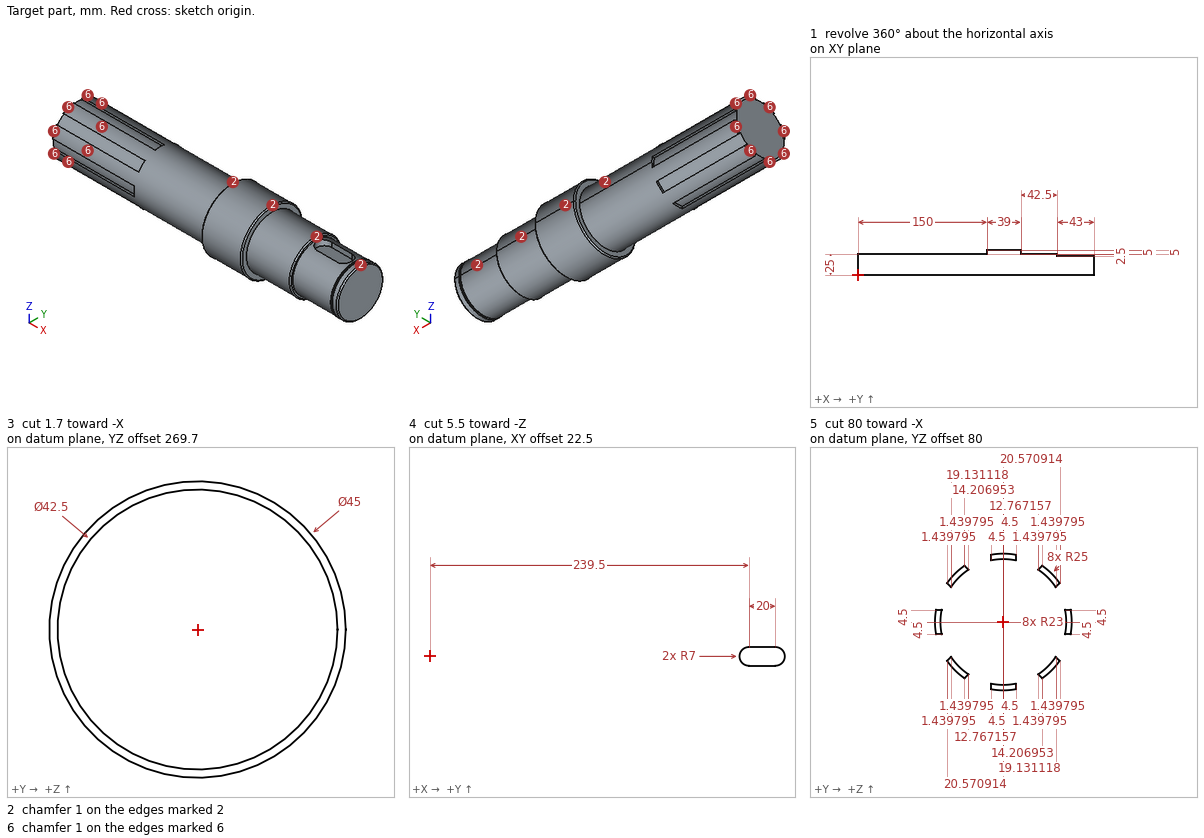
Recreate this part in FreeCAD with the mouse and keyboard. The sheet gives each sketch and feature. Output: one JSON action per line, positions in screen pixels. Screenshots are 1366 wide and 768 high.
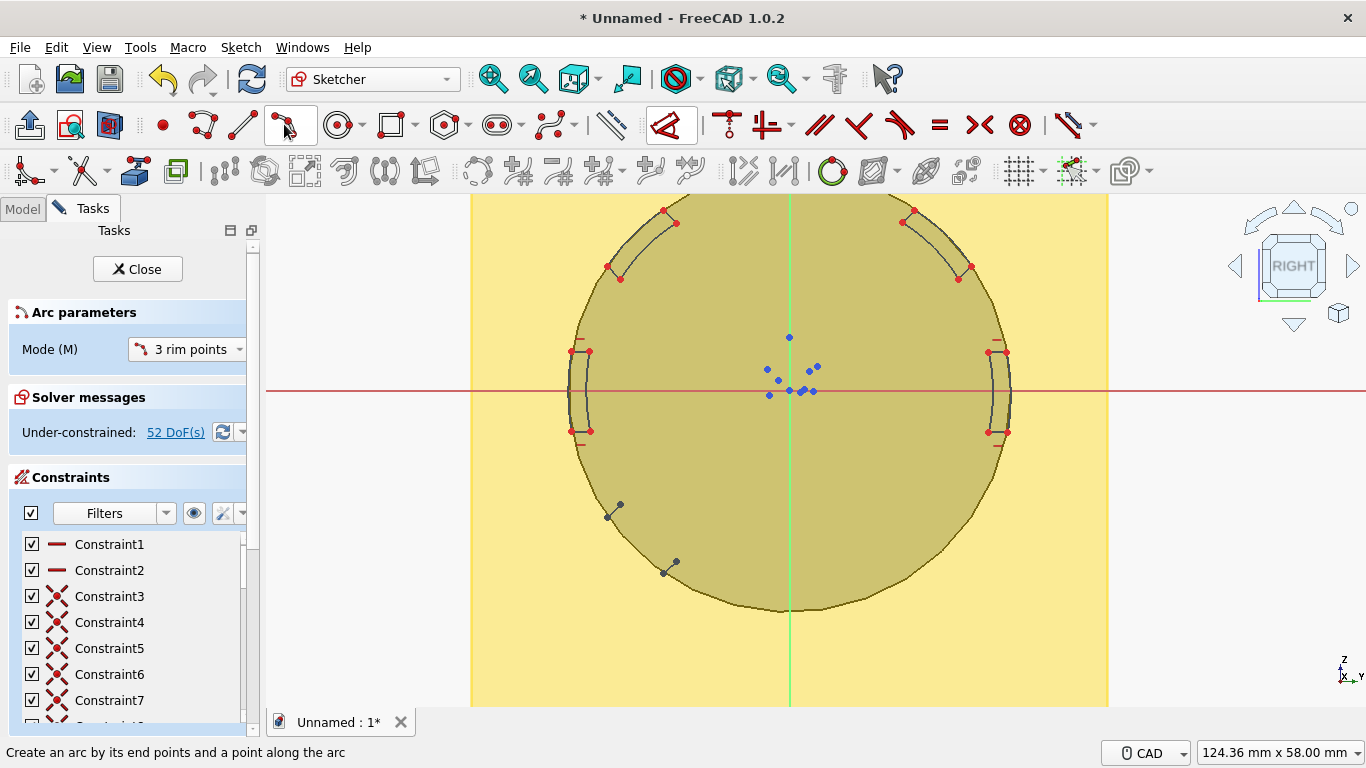
{"action": "scroll", "coordinate": [664, 573], "scroll_direction": "up", "scroll_amount": 3}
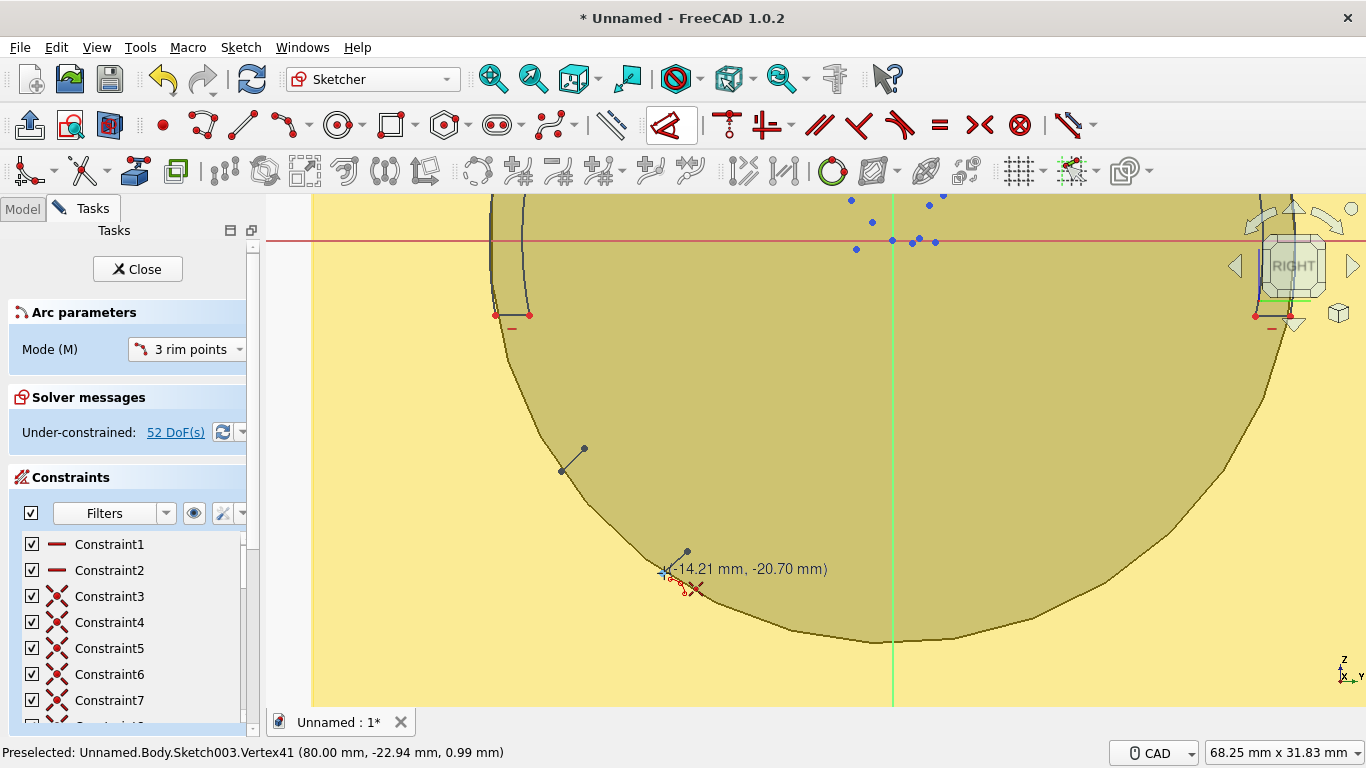
{"action": "left_click", "coordinate": [663, 573]}
{"action": "left_click", "coordinate": [561, 472]}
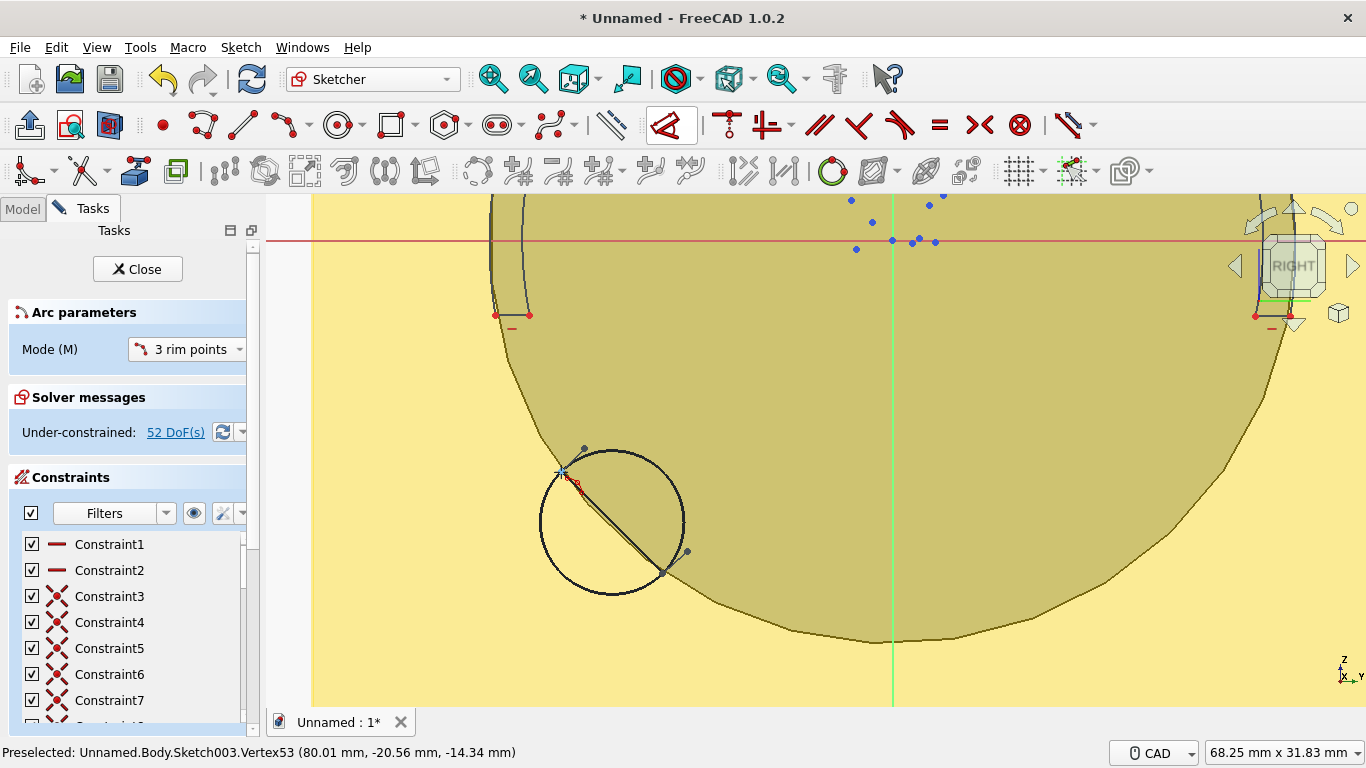
{"action": "scroll", "coordinate": [608, 526], "scroll_direction": "up", "scroll_amount": 5}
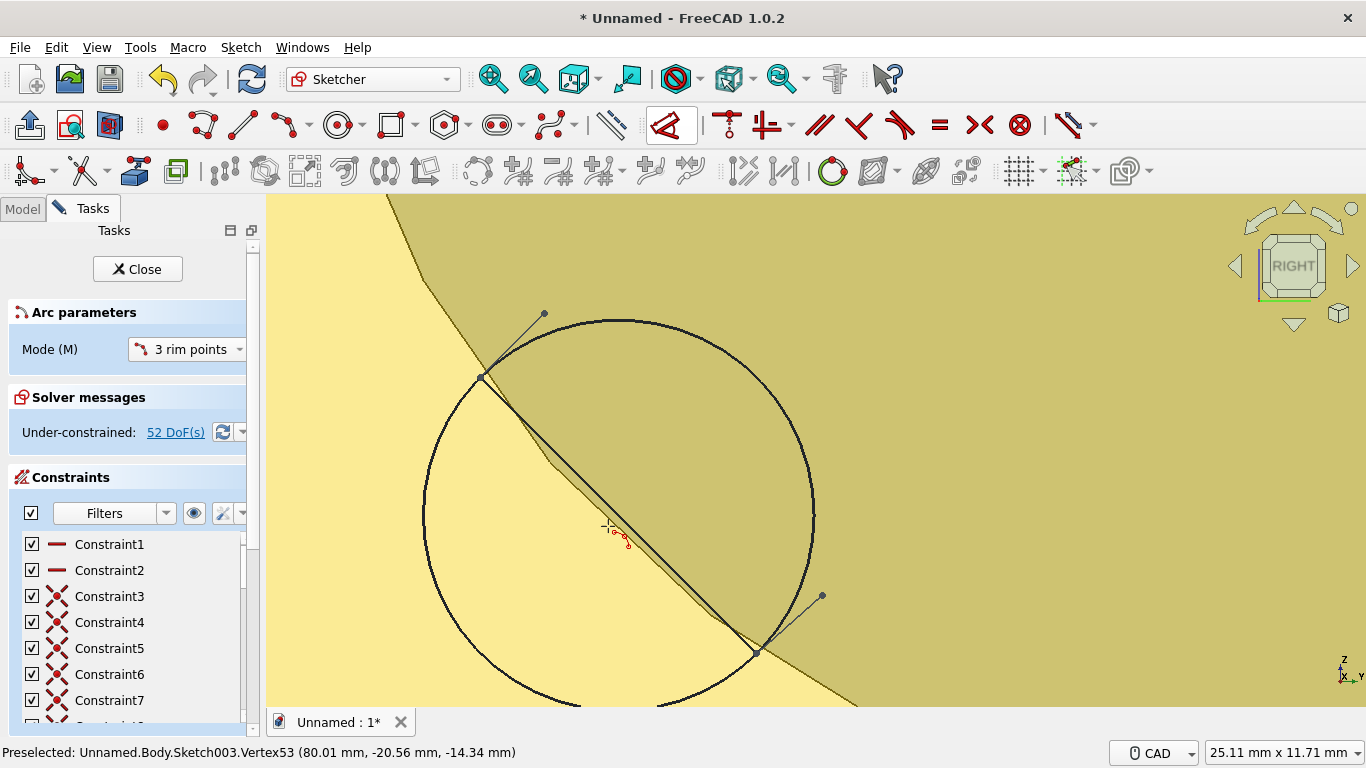
{"action": "left_click", "coordinate": [607, 524]}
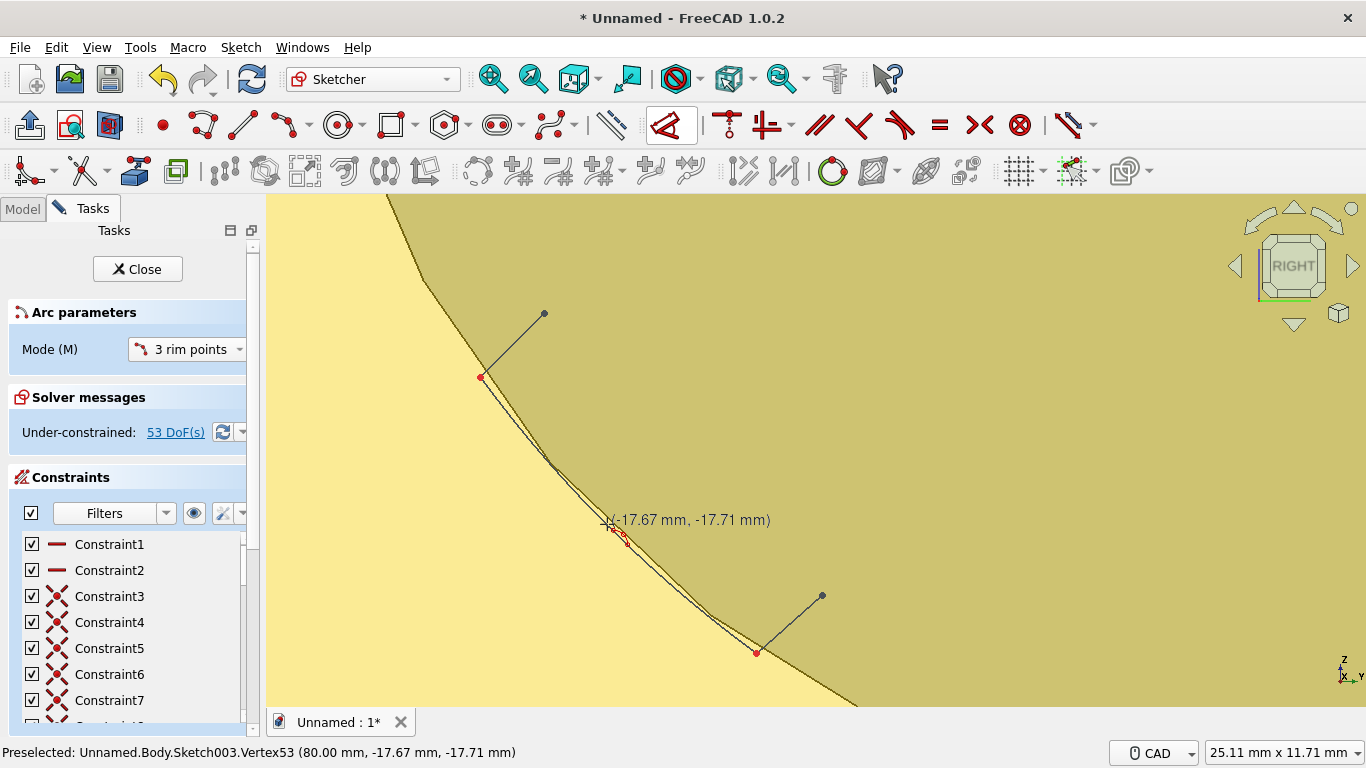
{"action": "left_click", "coordinate": [545, 313]}
{"action": "left_click", "coordinate": [822, 595]}
{"action": "left_click", "coordinate": [669, 462]}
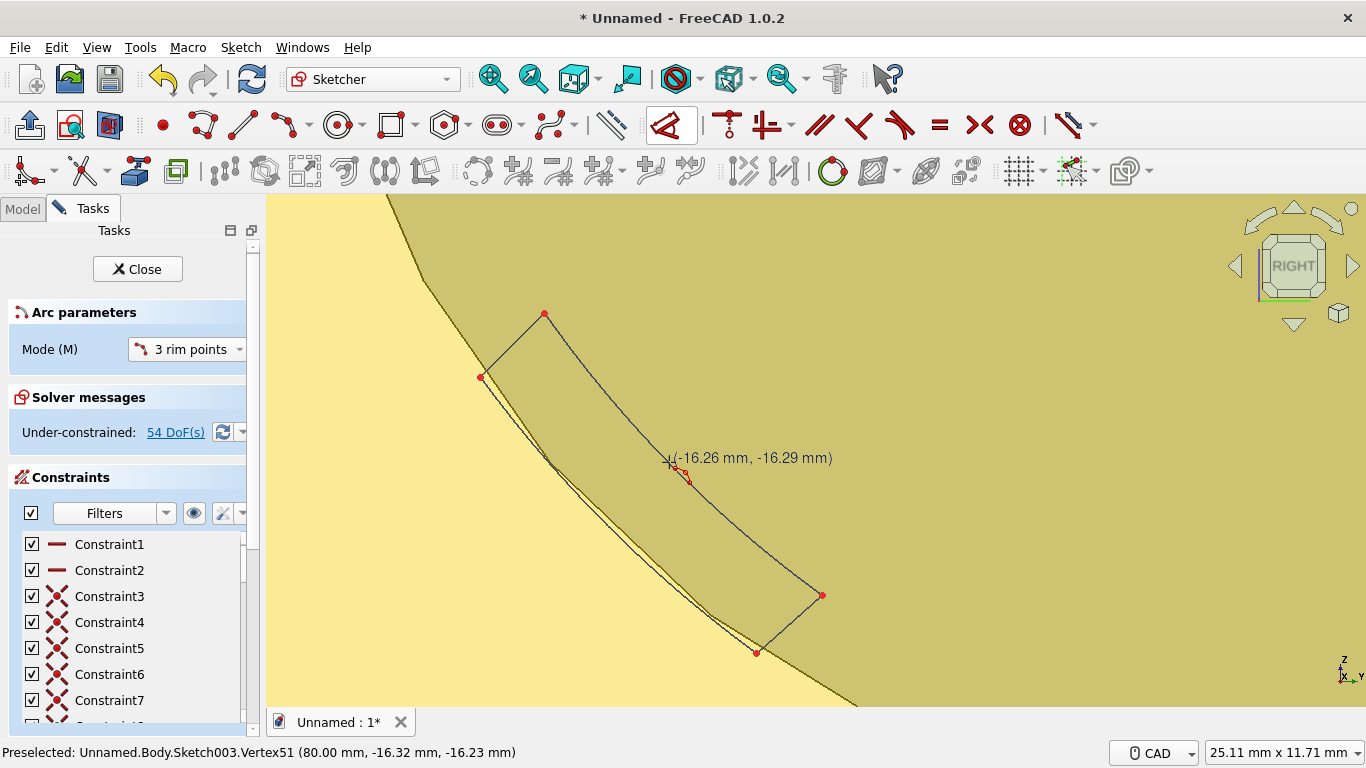
{"action": "left_click", "coordinate": [244, 126]}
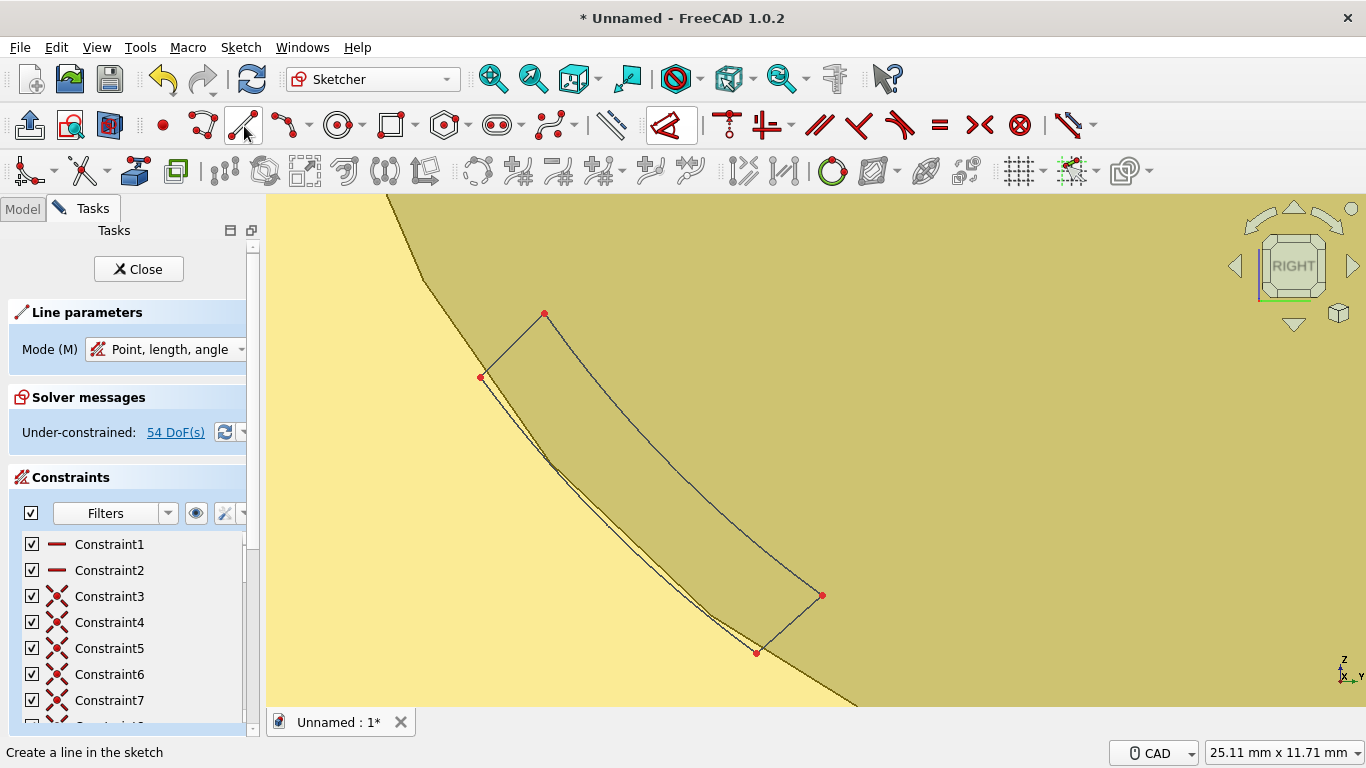
{"action": "scroll", "coordinate": [648, 560], "scroll_direction": "down", "scroll_amount": 10}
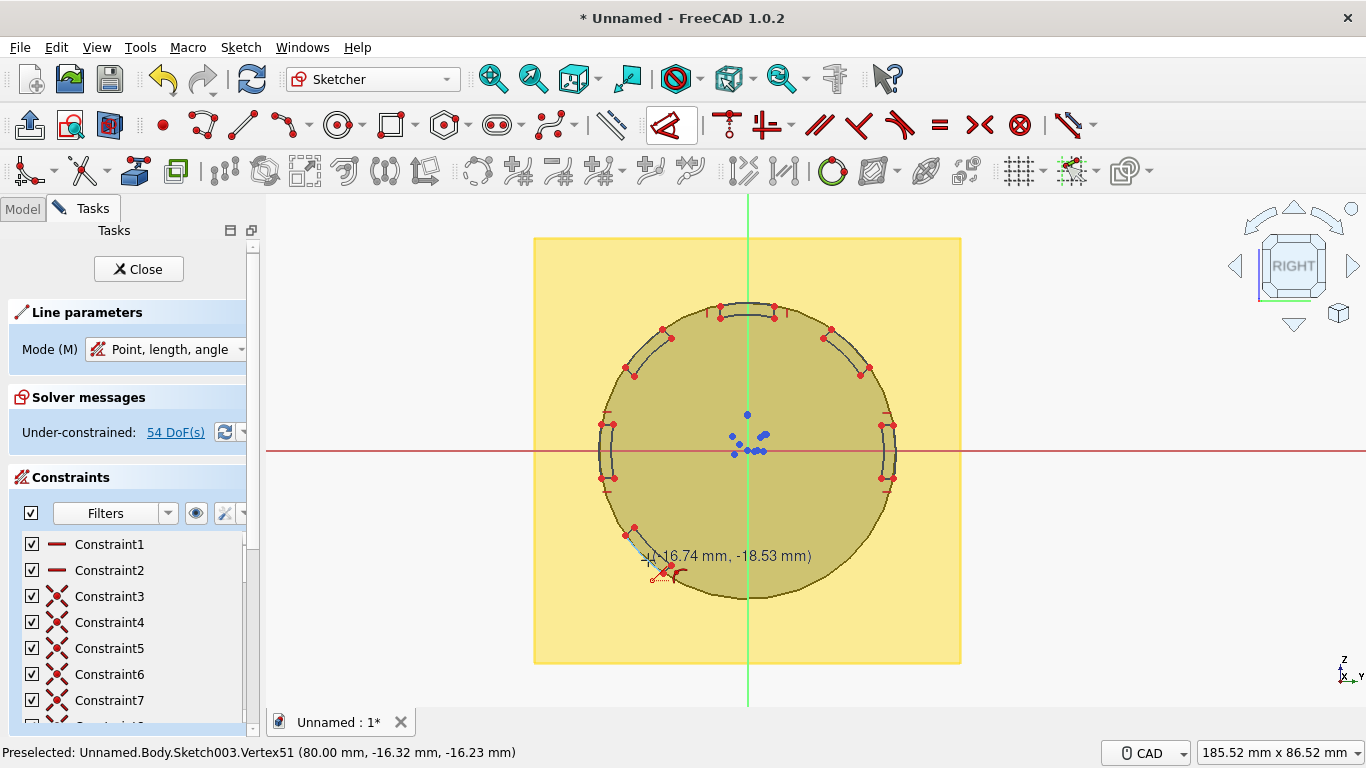
{"action": "left_click", "coordinate": [774, 585]}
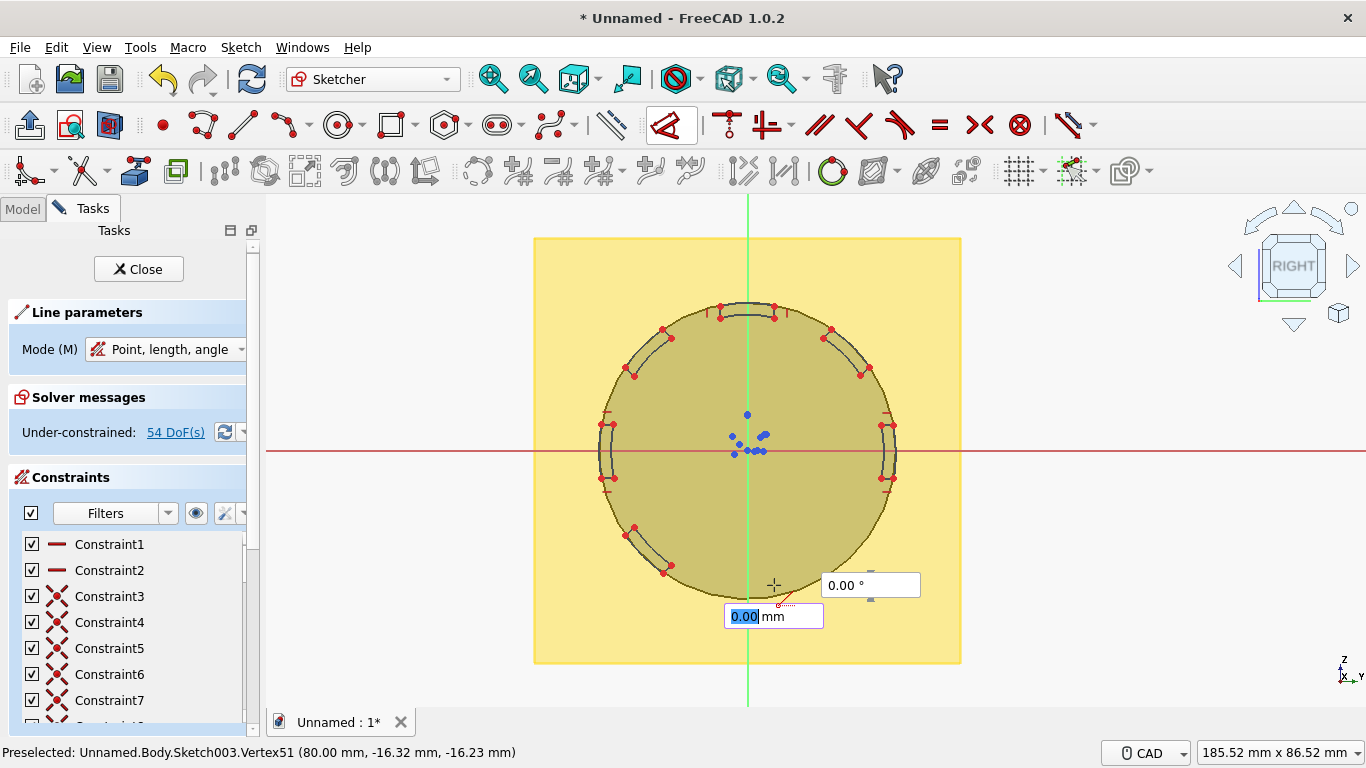
{"action": "scroll", "coordinate": [774, 597], "scroll_direction": "up", "scroll_amount": 2}